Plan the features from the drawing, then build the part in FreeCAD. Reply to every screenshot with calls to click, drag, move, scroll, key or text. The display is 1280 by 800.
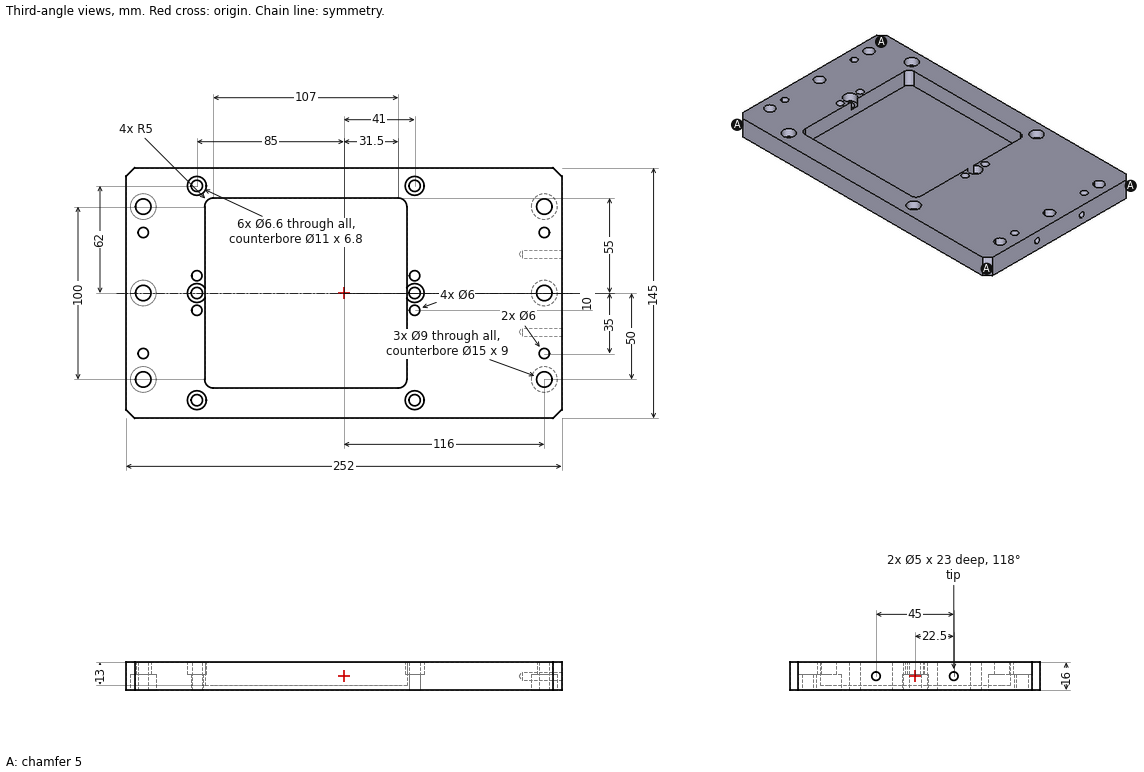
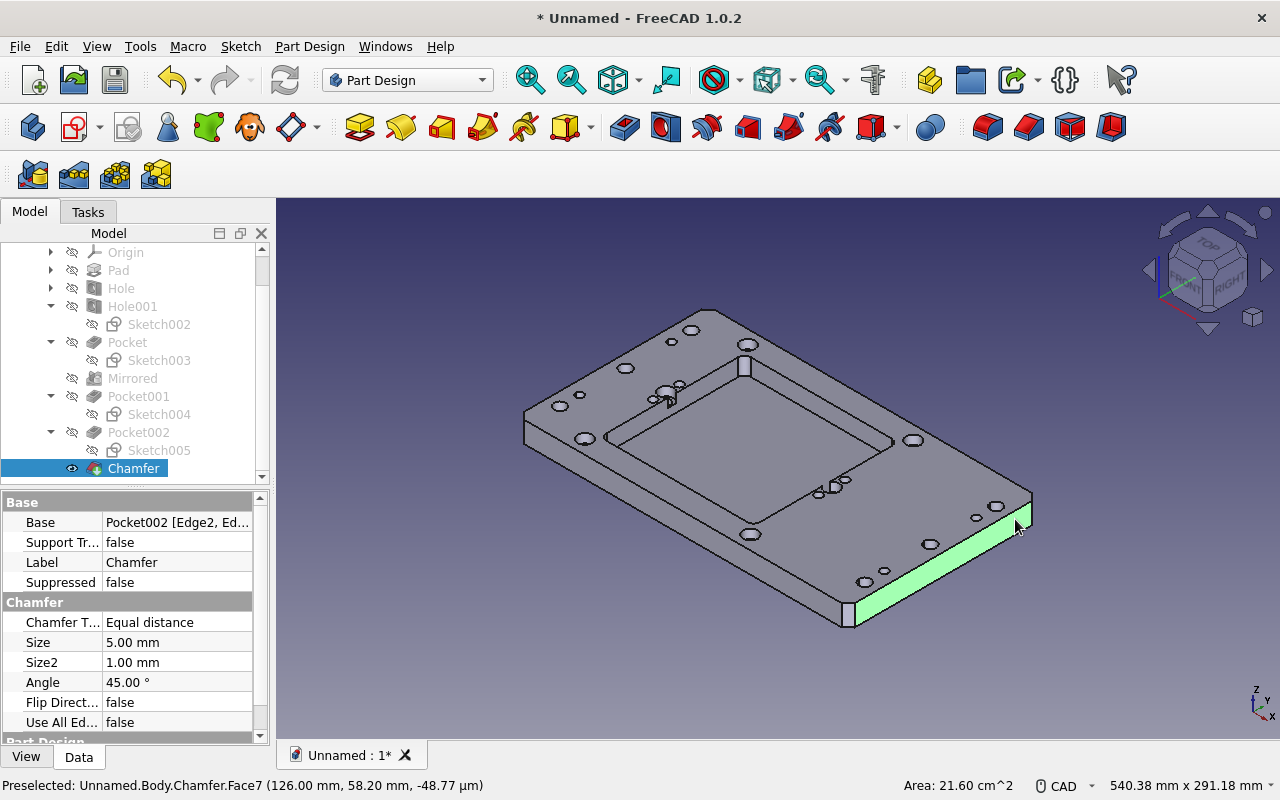
click(74, 128)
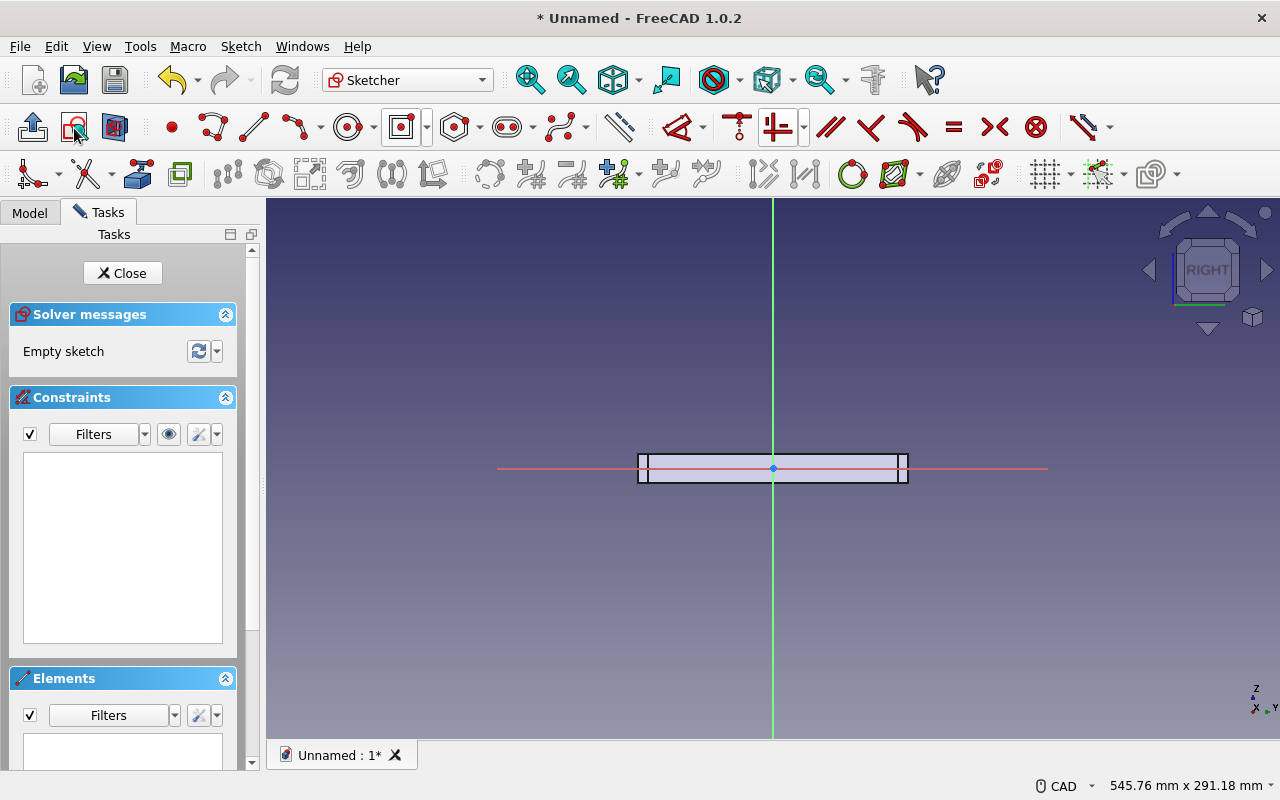
scroll(787, 468, up, 9)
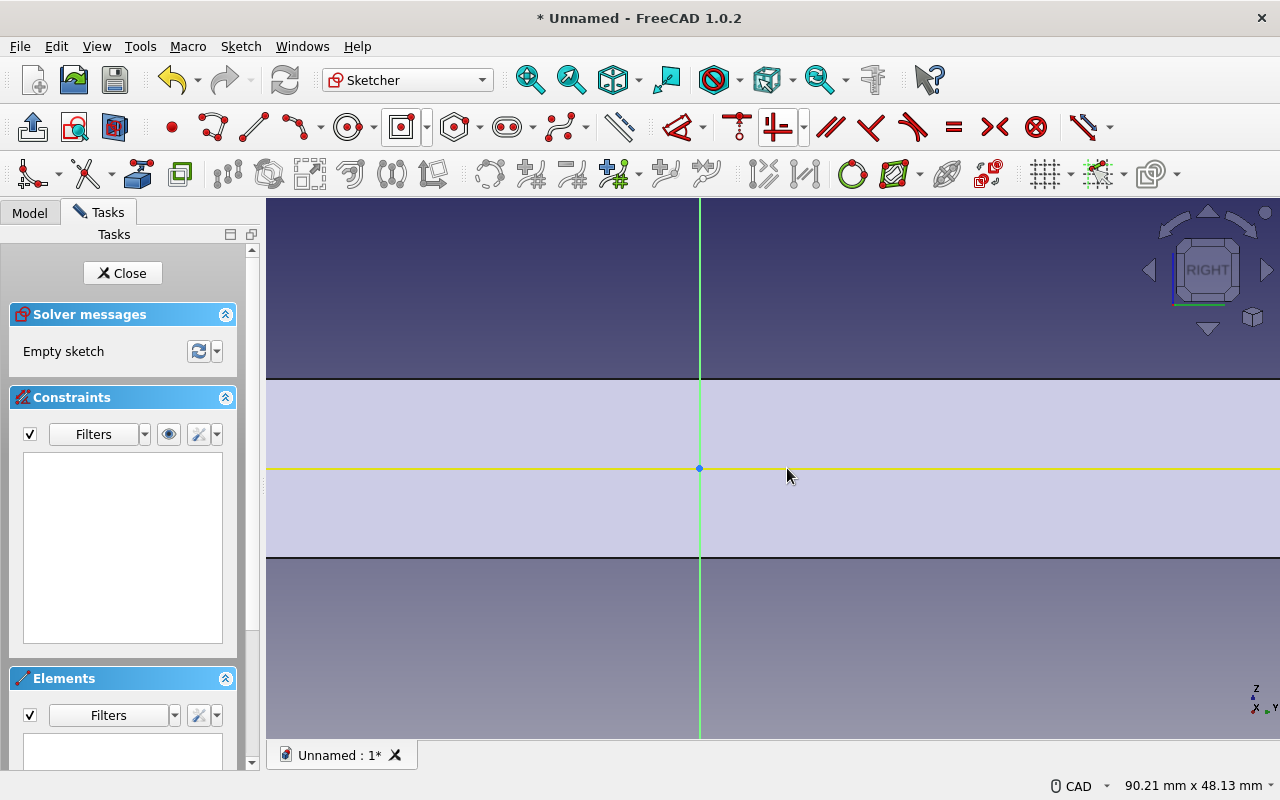
key(g)
key(c)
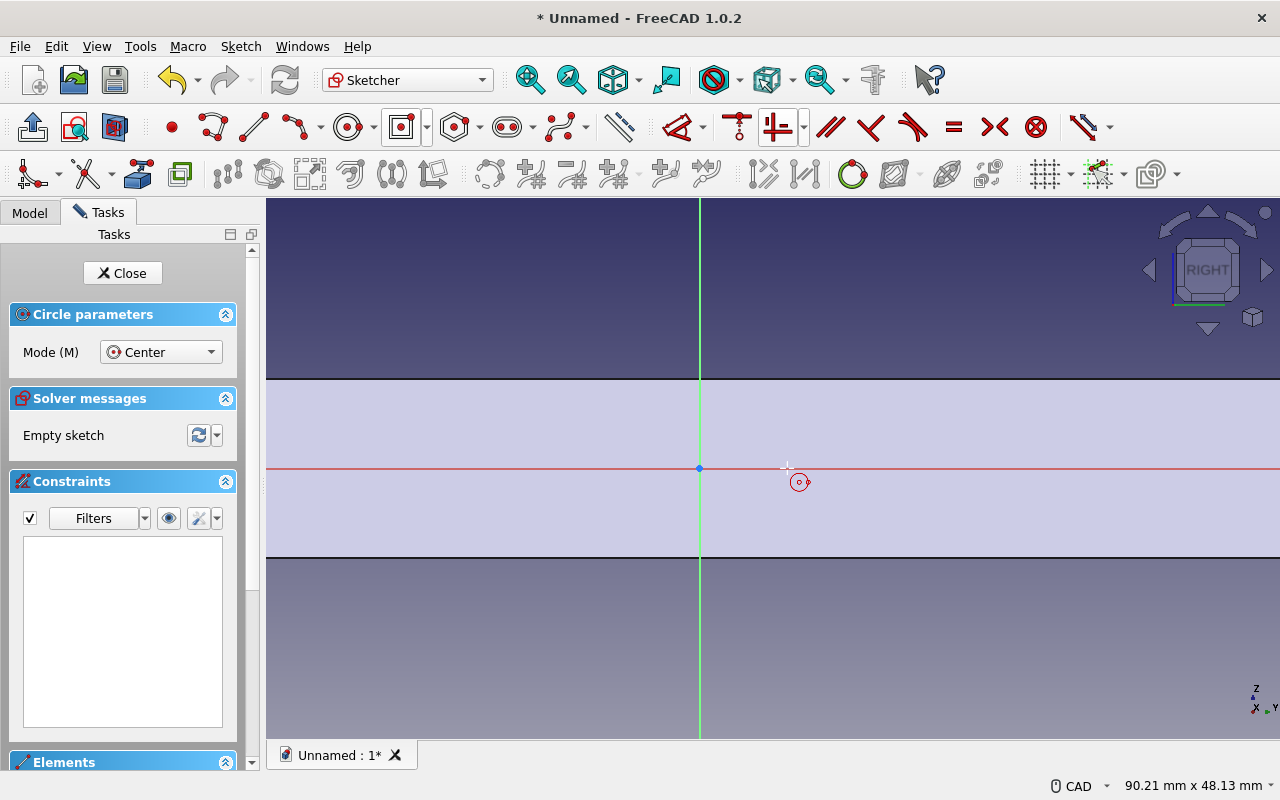
click(953, 468)
move(972, 449)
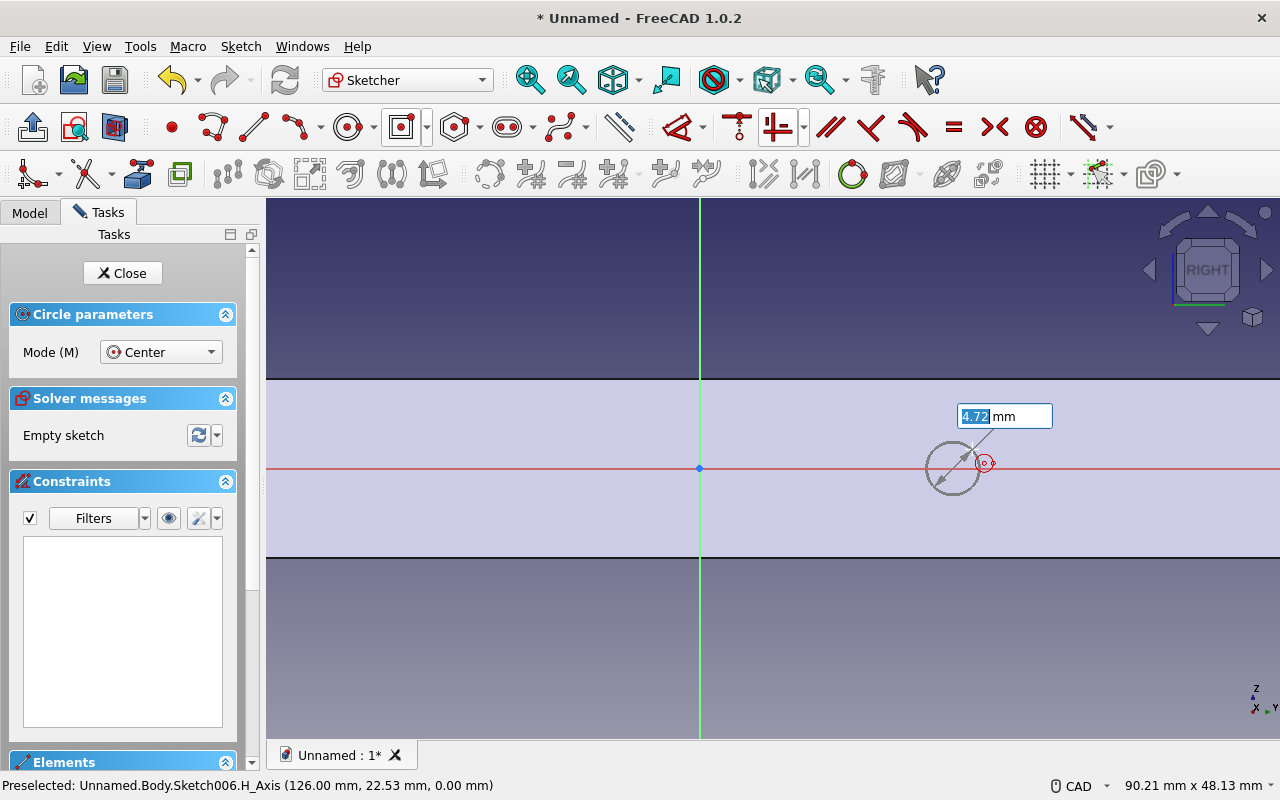
text(5)
key(Return)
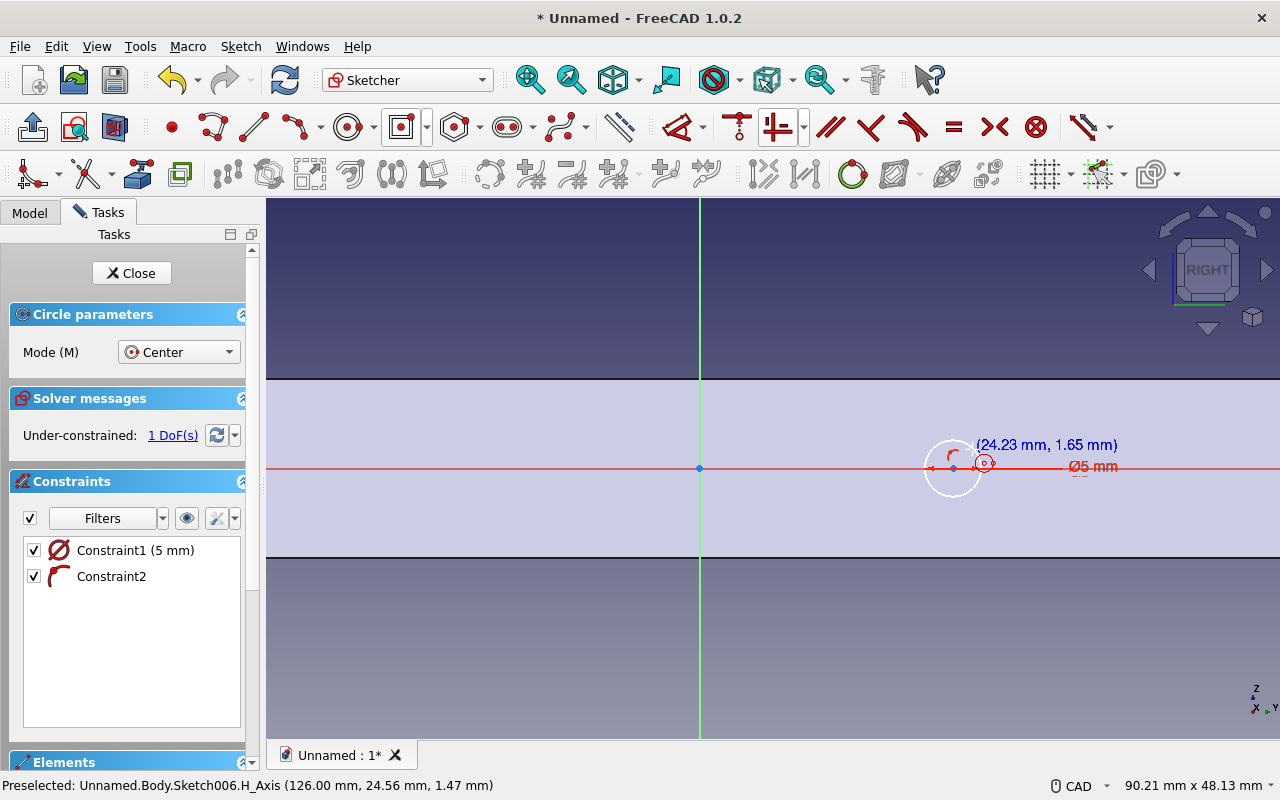
click(447, 468)
move(467, 449)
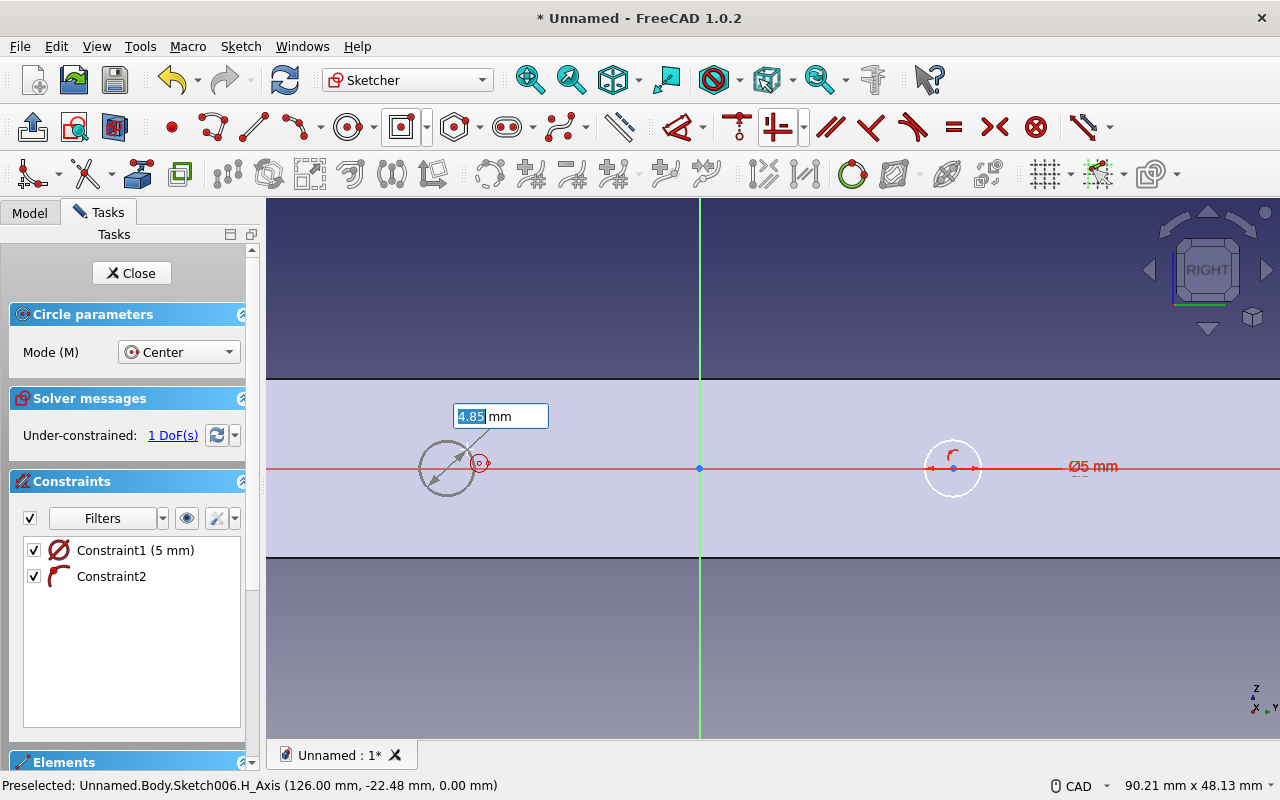
text(5)
key(Return)
key(Escape)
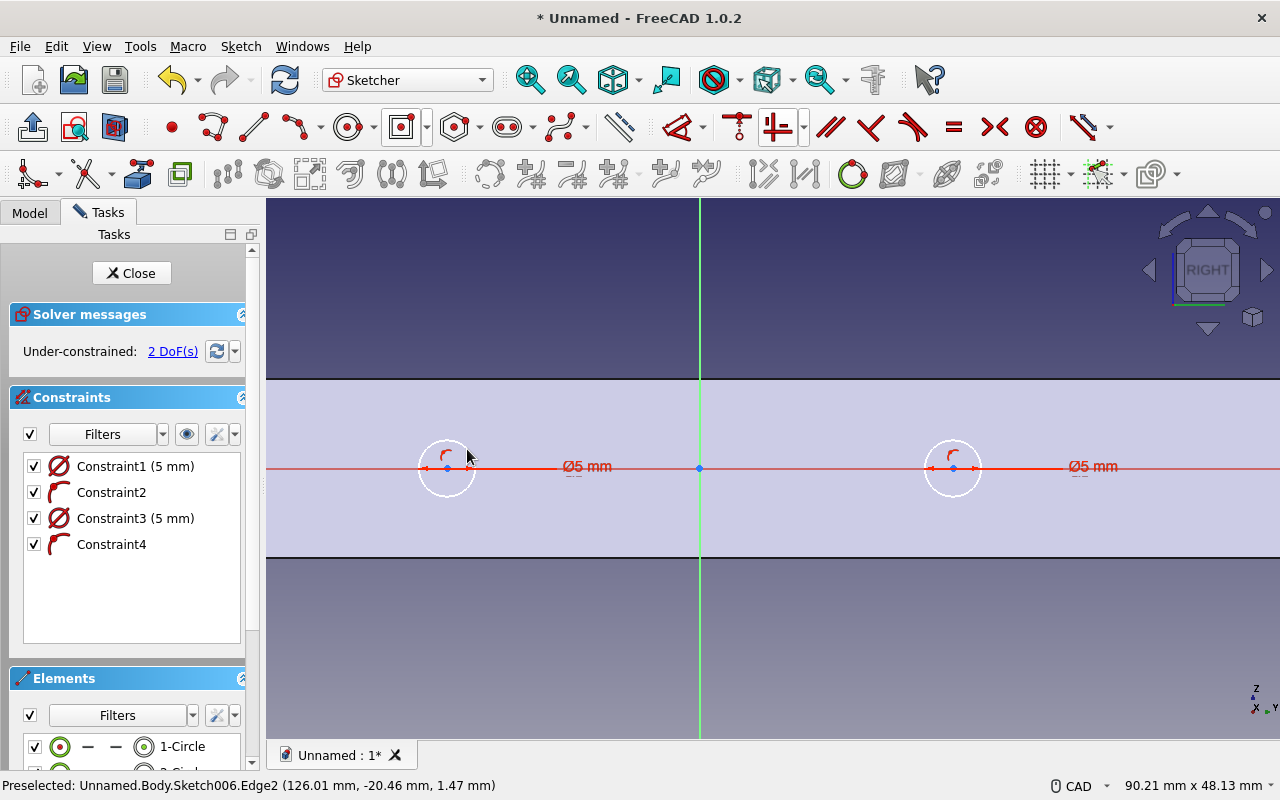
key(d)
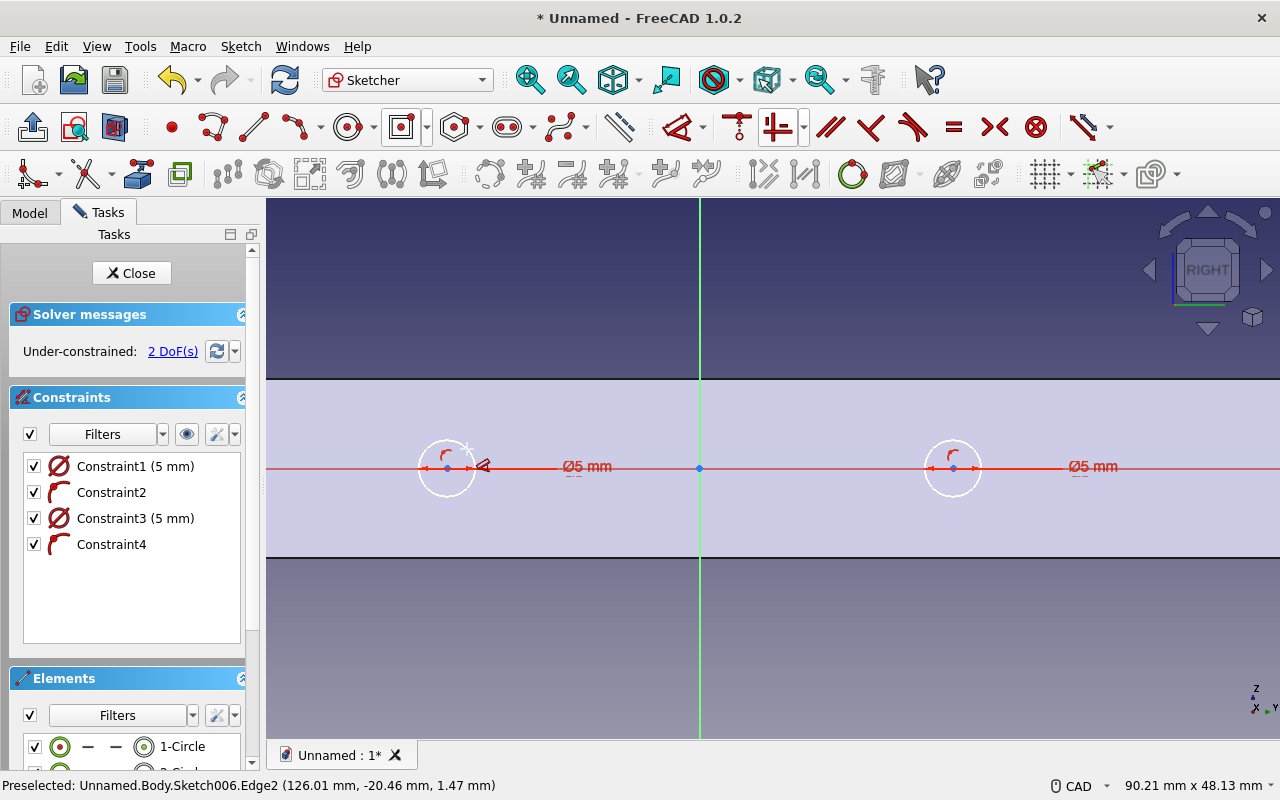
click(953, 468)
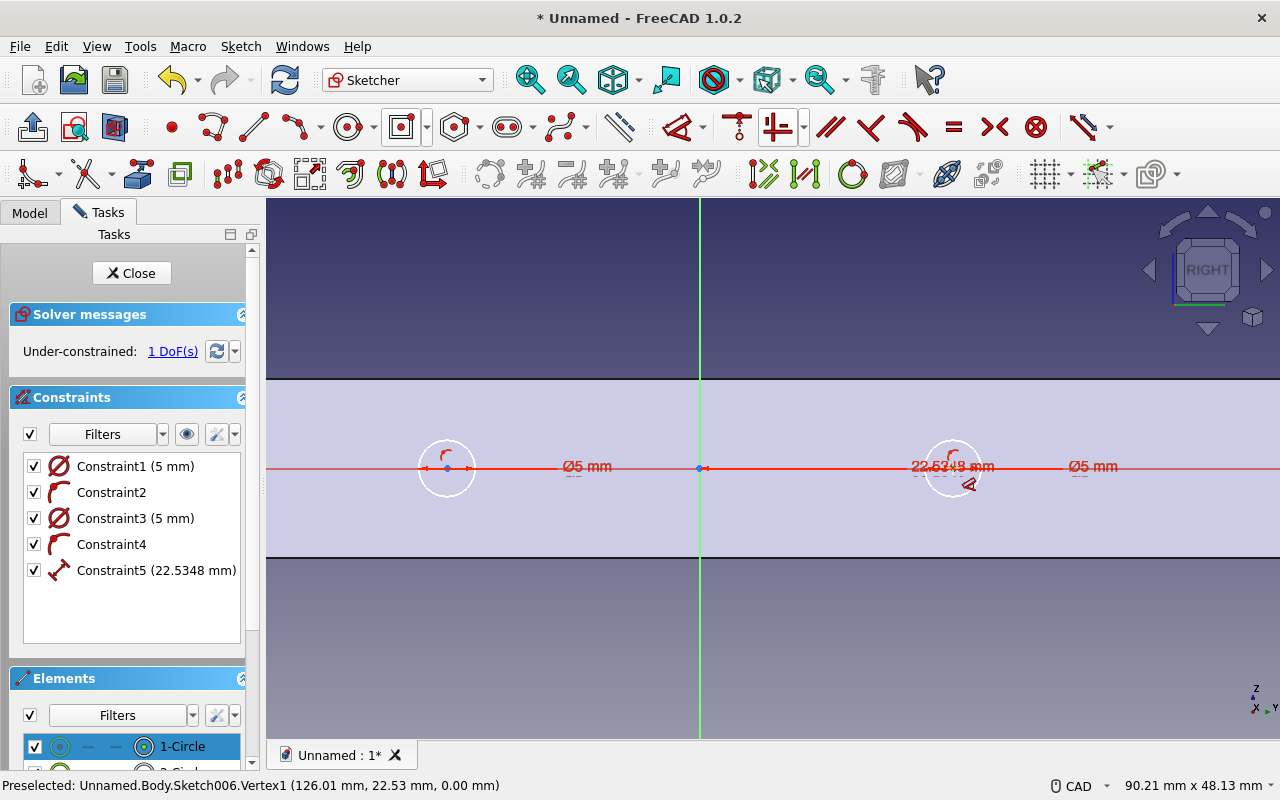
click(447, 468)
click(584, 502)